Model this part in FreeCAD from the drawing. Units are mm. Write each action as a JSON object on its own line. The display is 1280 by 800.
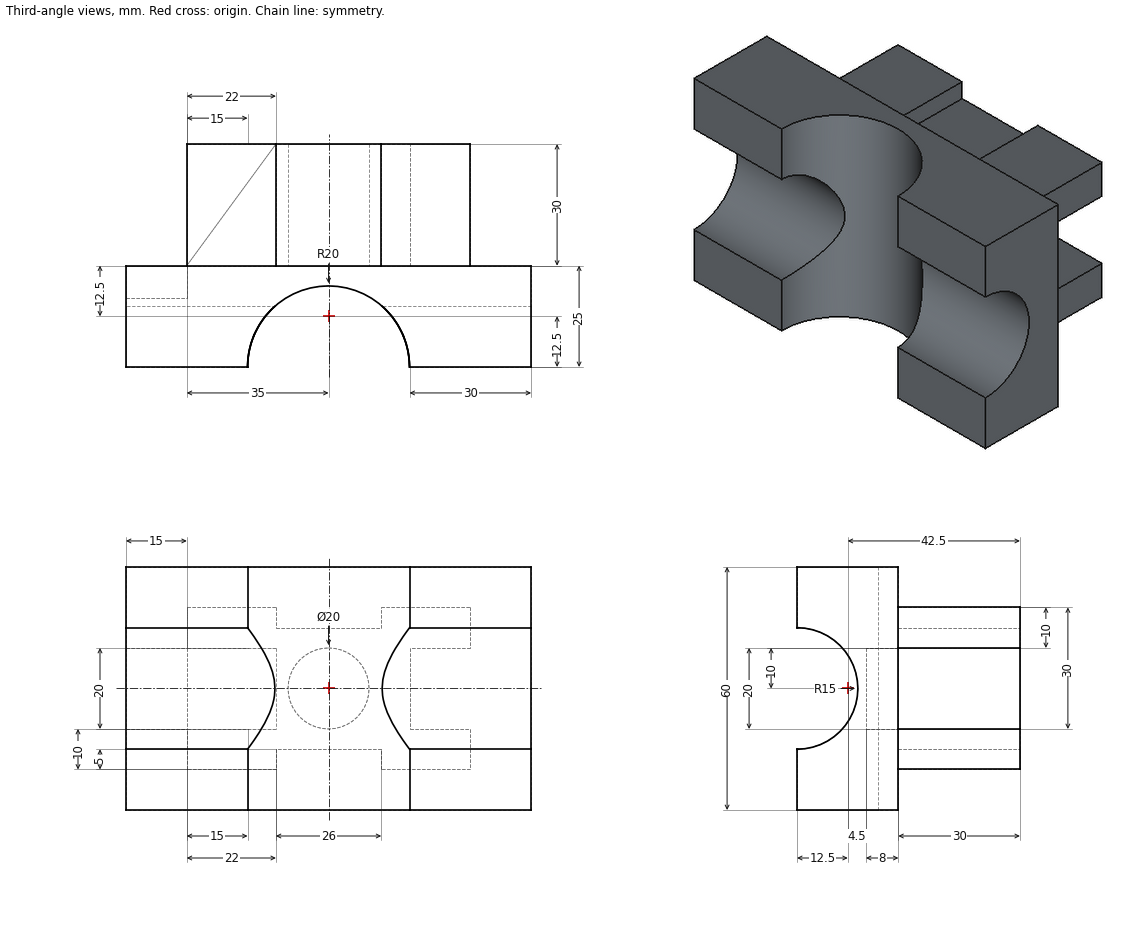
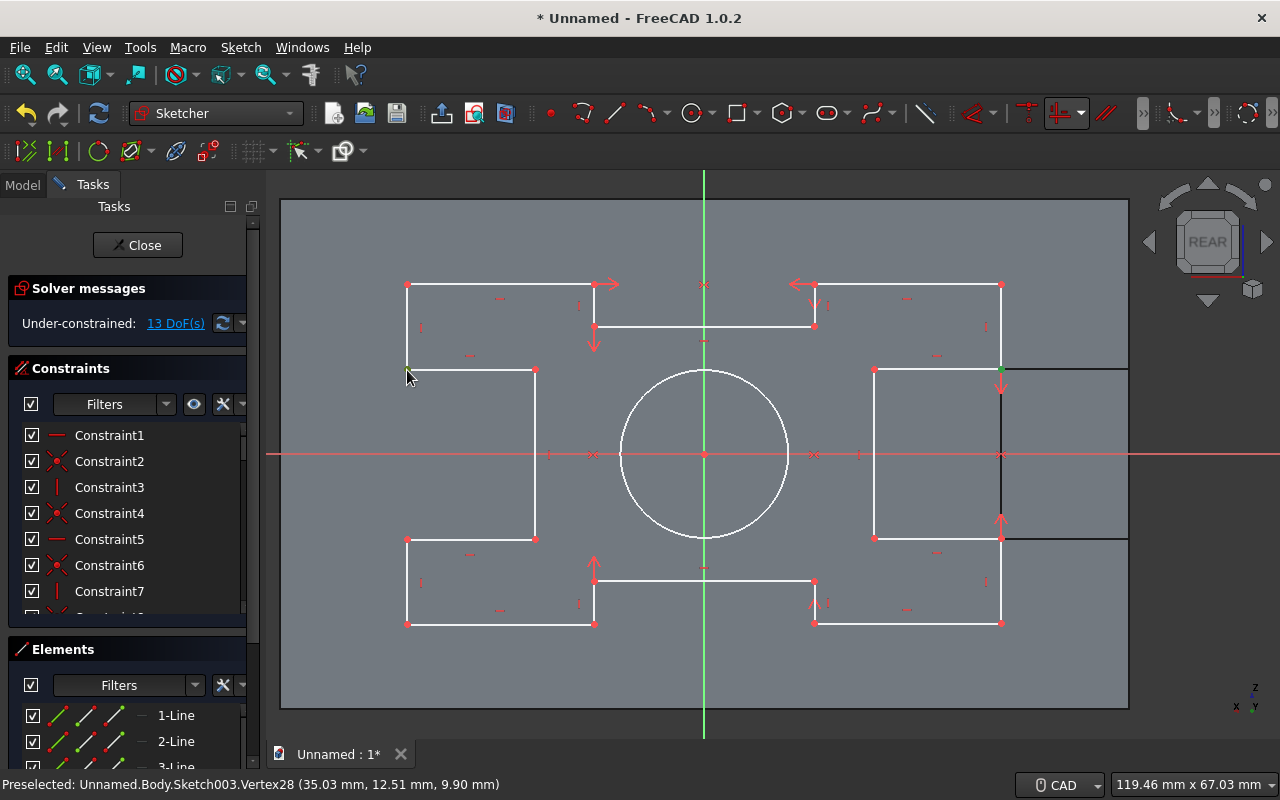
{"action": "left_click", "coordinate": [704, 674]}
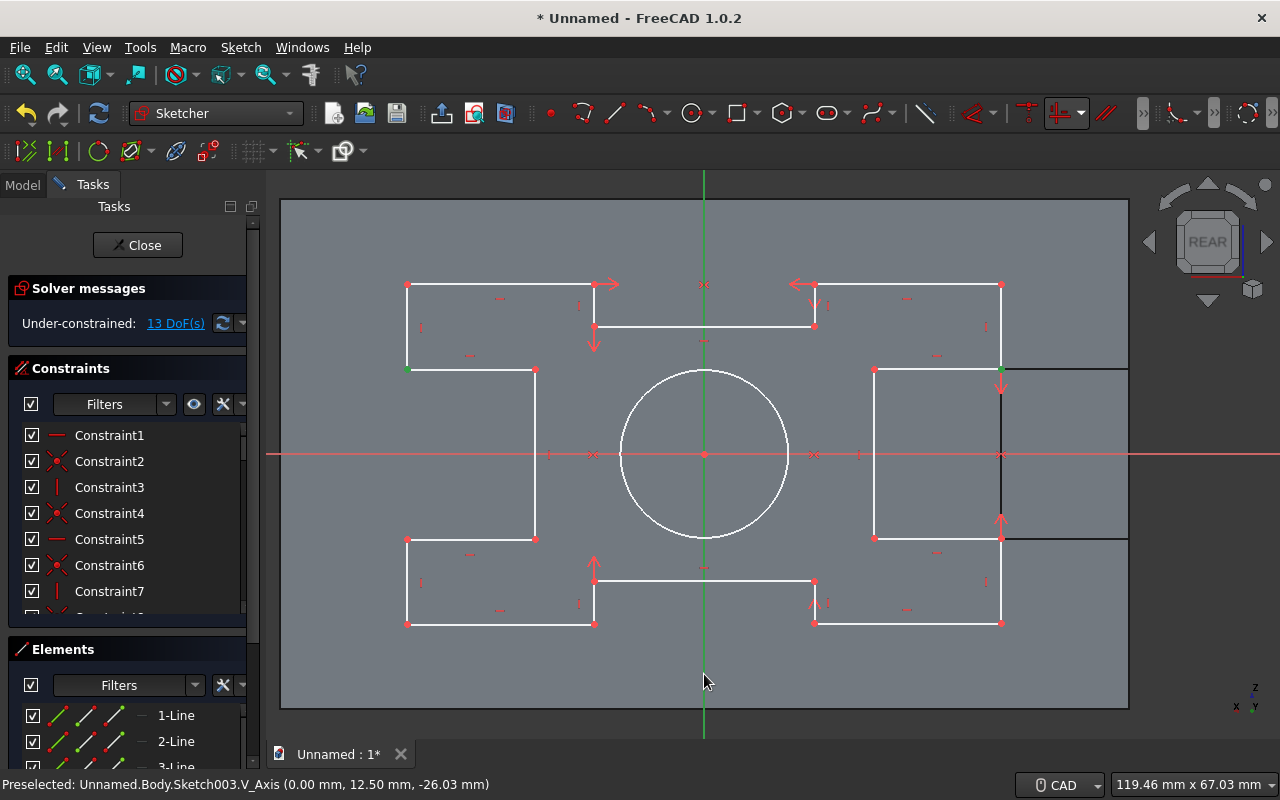
{"action": "key", "text": "s"}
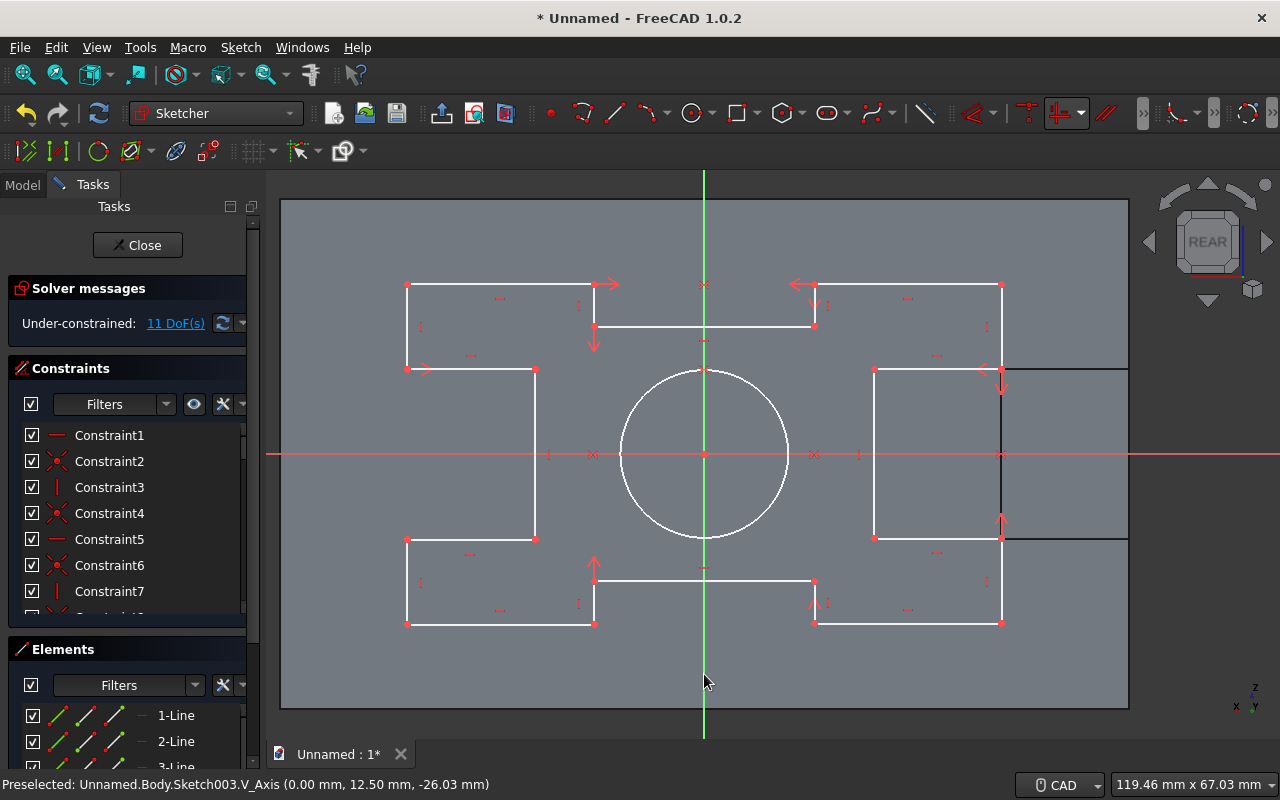
{"action": "left_click", "coordinate": [874, 539]}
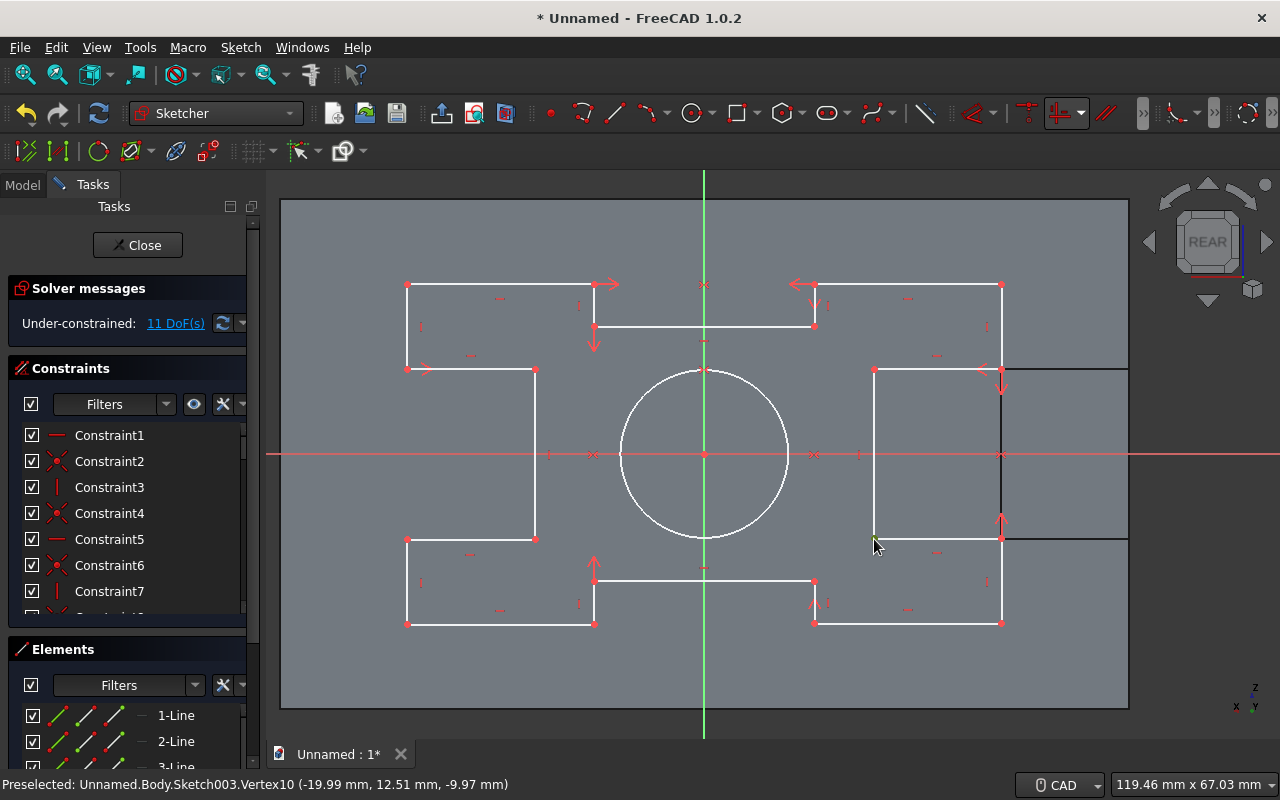
{"action": "left_click", "coordinate": [535, 540]}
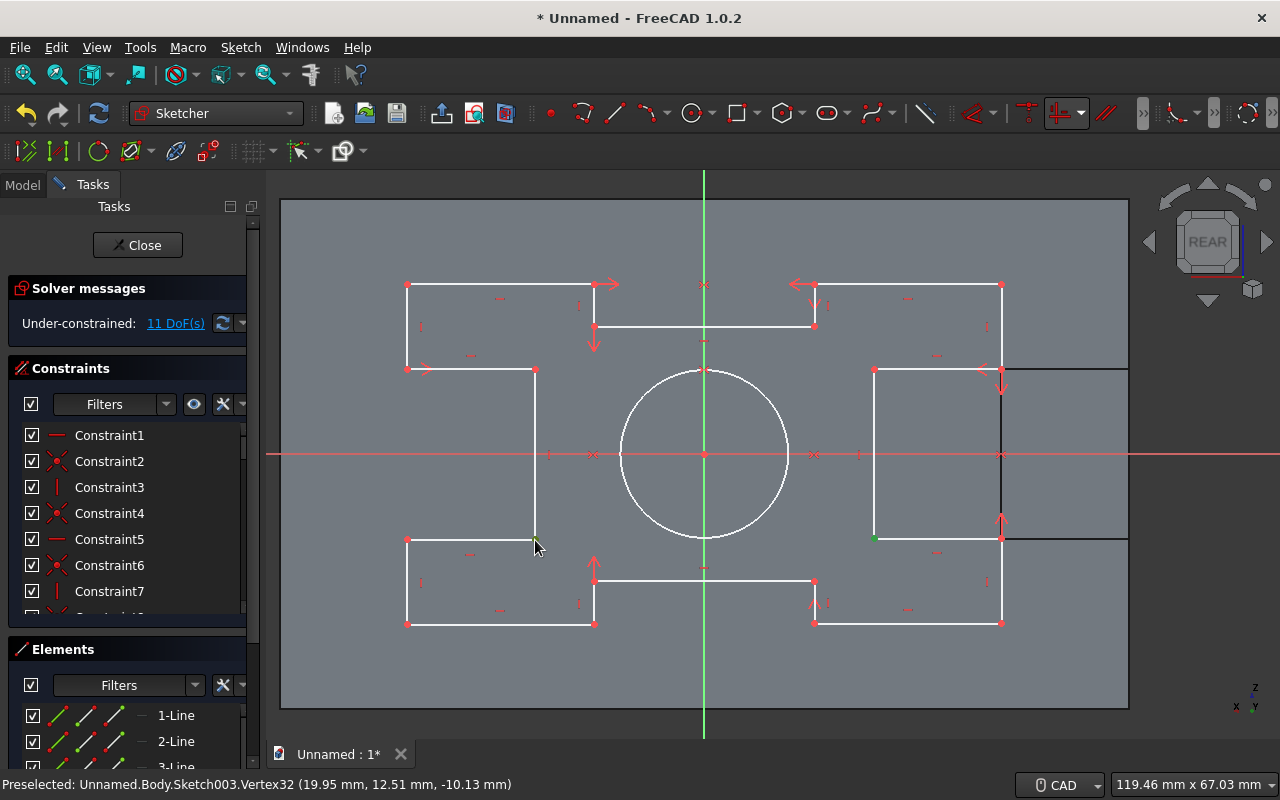
{"action": "left_click", "coordinate": [704, 674]}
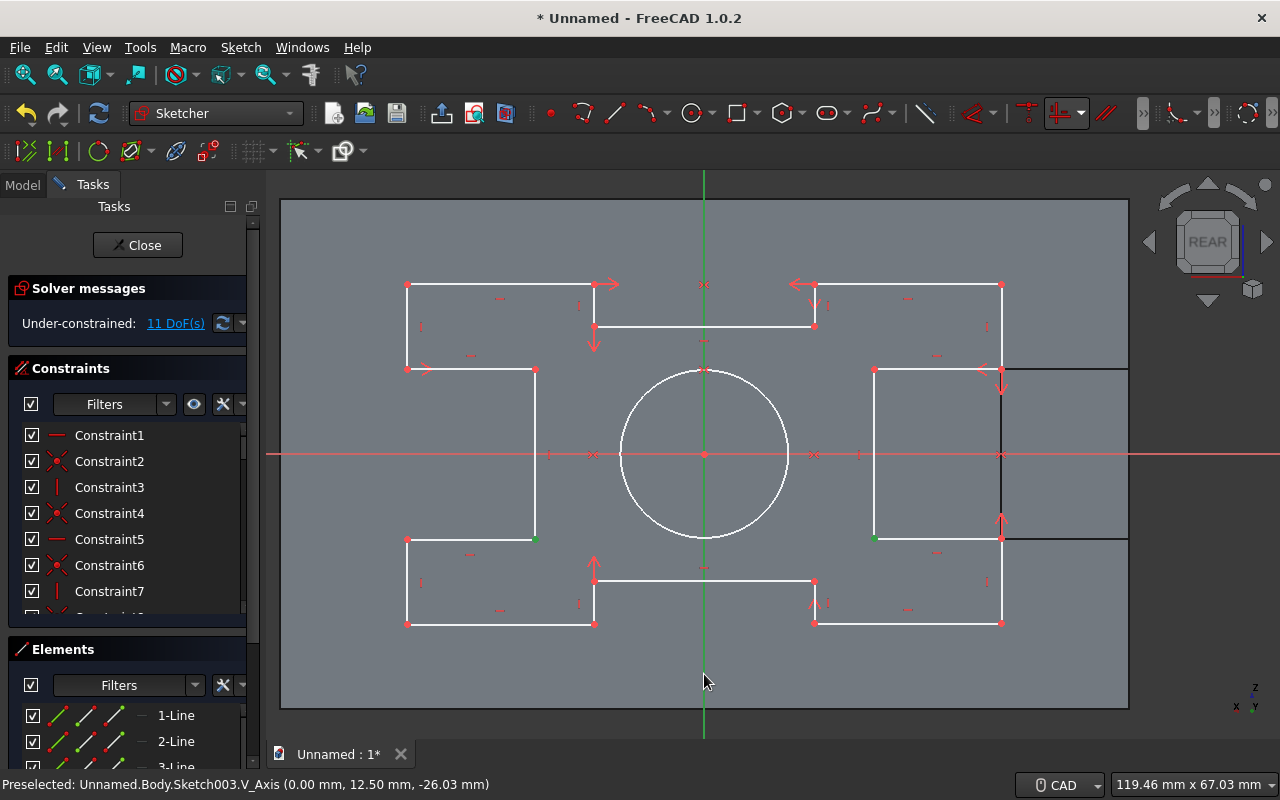
{"action": "key", "text": "s"}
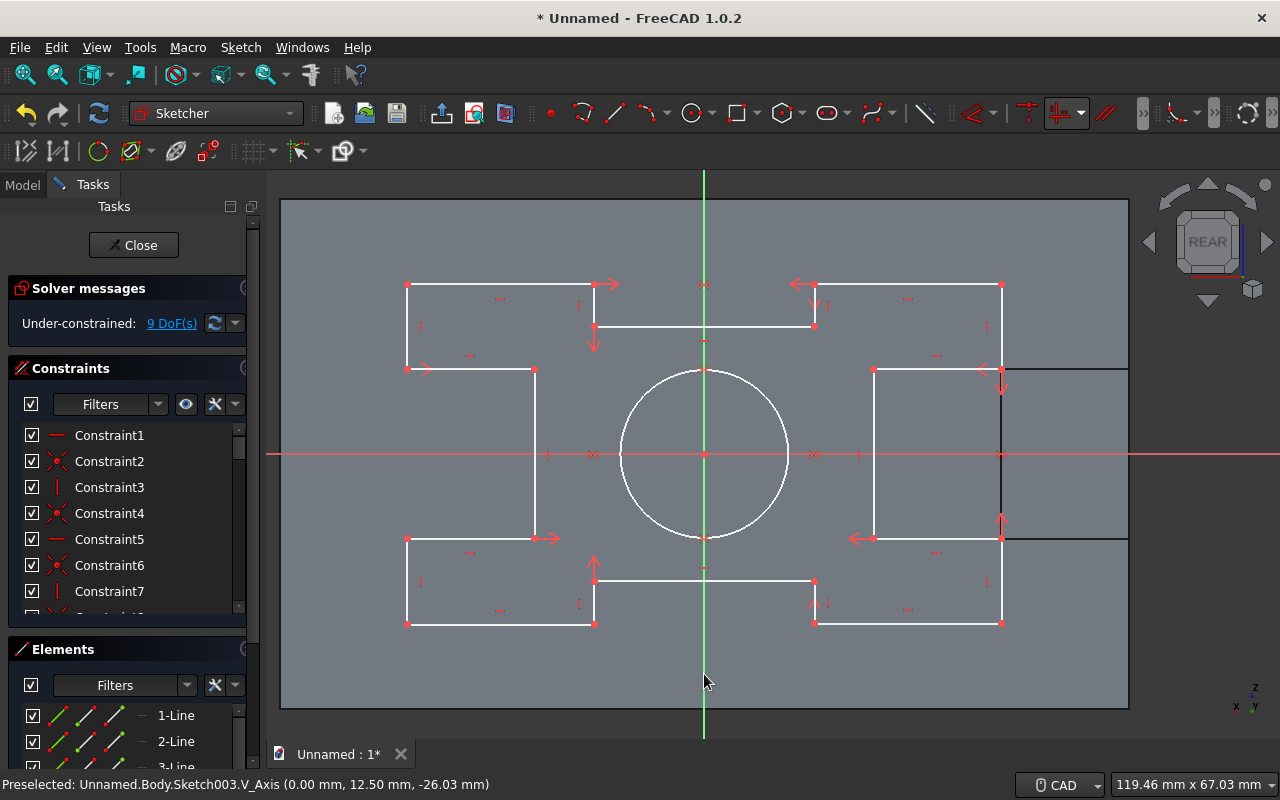
{"action": "left_click", "coordinate": [1002, 624]}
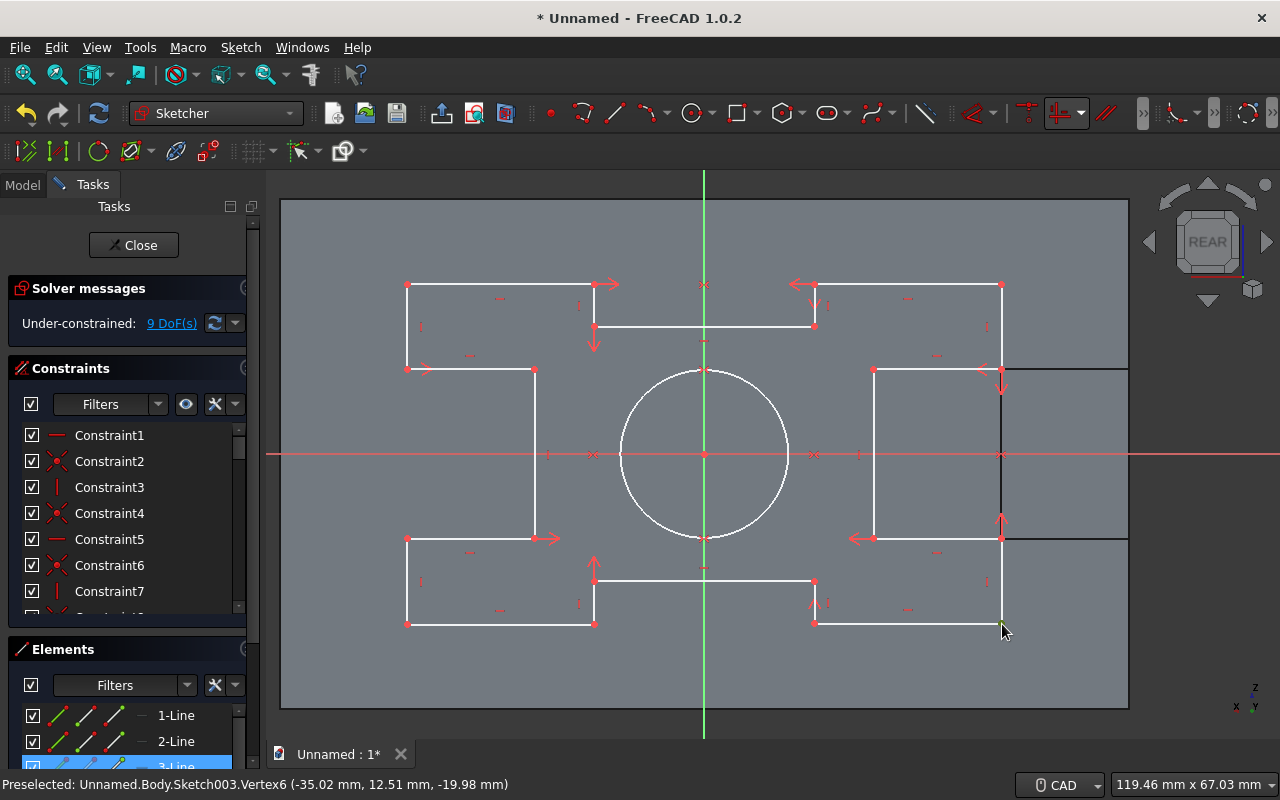
{"action": "left_click", "coordinate": [407, 625]}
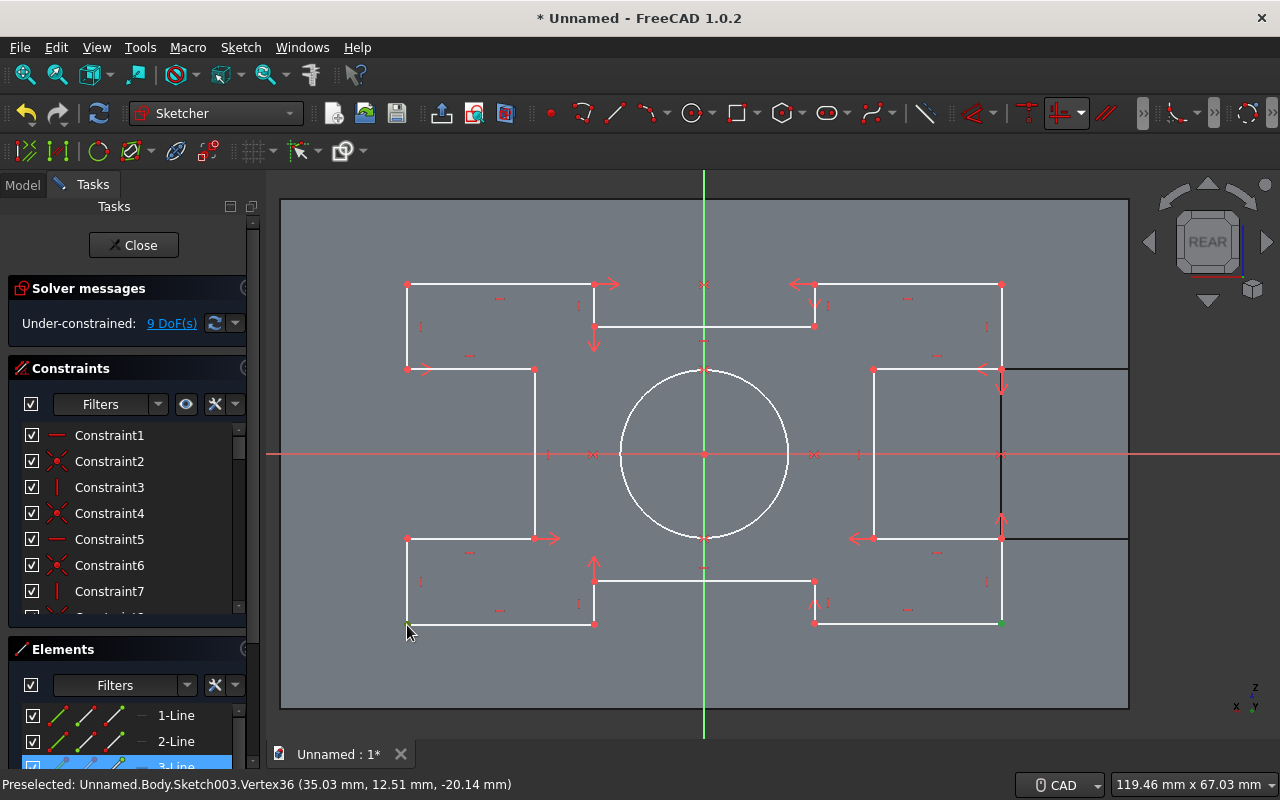
{"action": "left_click", "coordinate": [704, 674]}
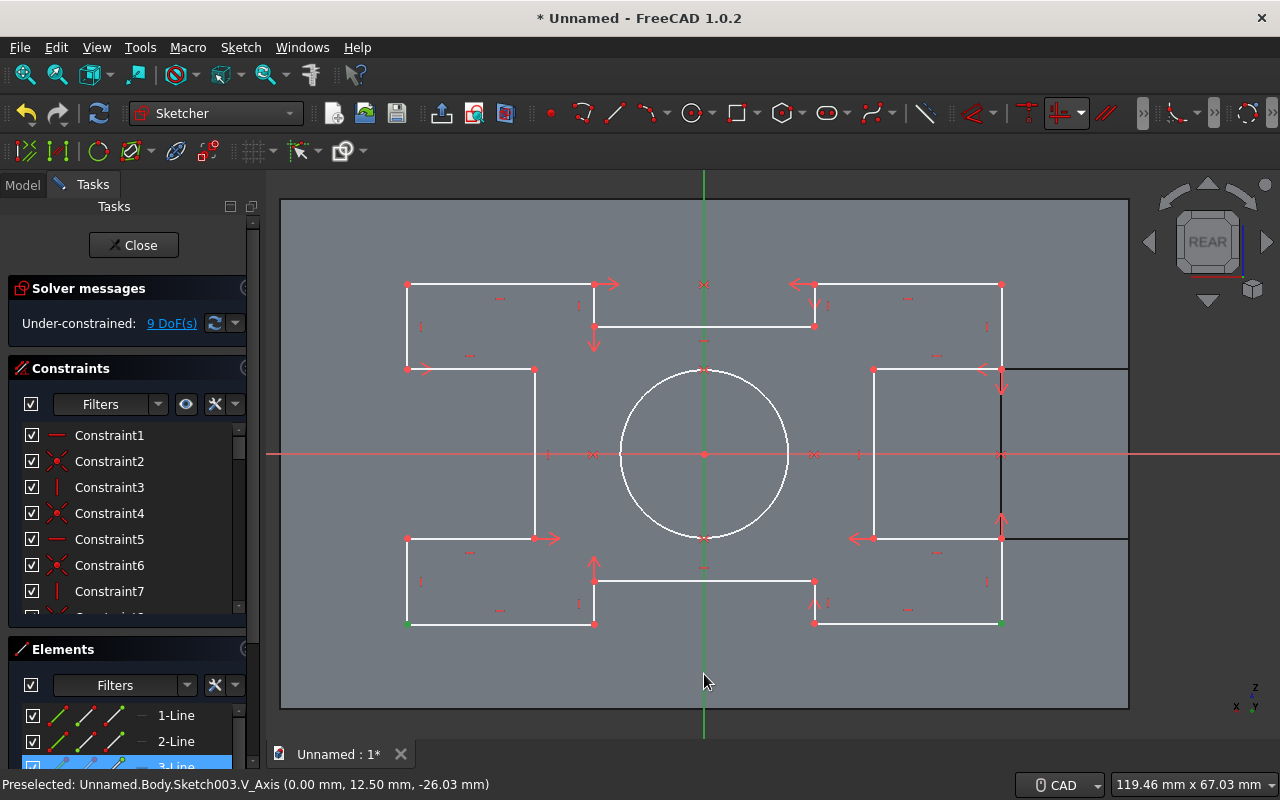
{"action": "key", "text": "s"}